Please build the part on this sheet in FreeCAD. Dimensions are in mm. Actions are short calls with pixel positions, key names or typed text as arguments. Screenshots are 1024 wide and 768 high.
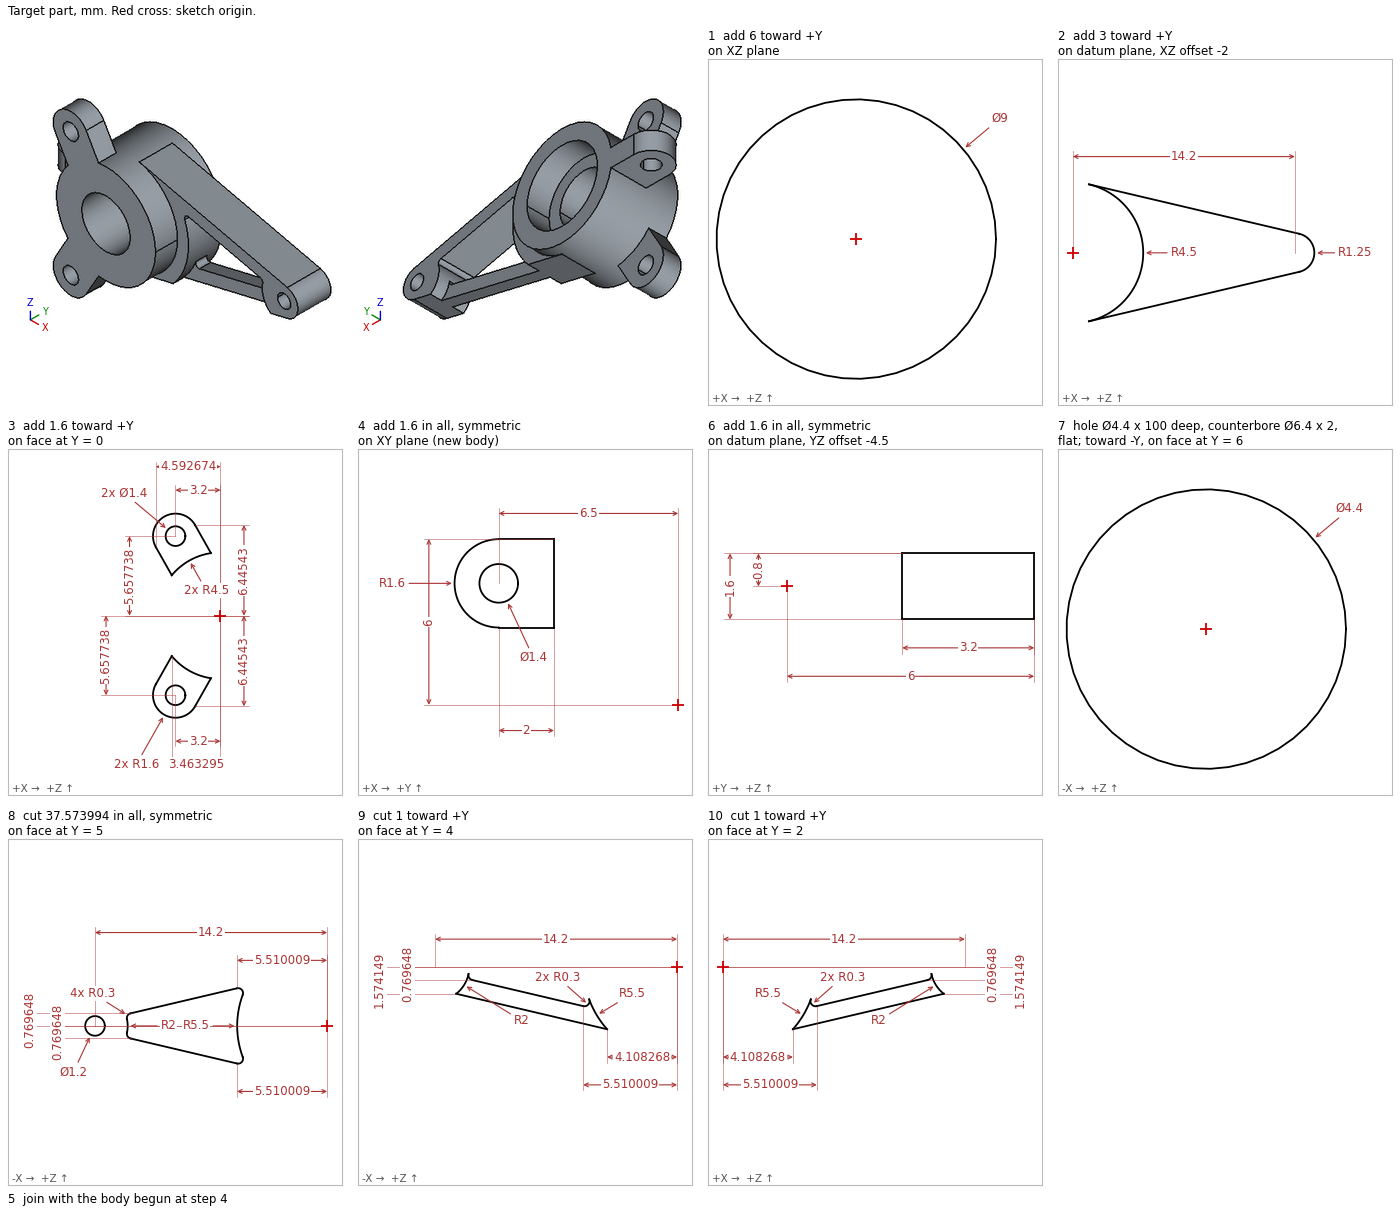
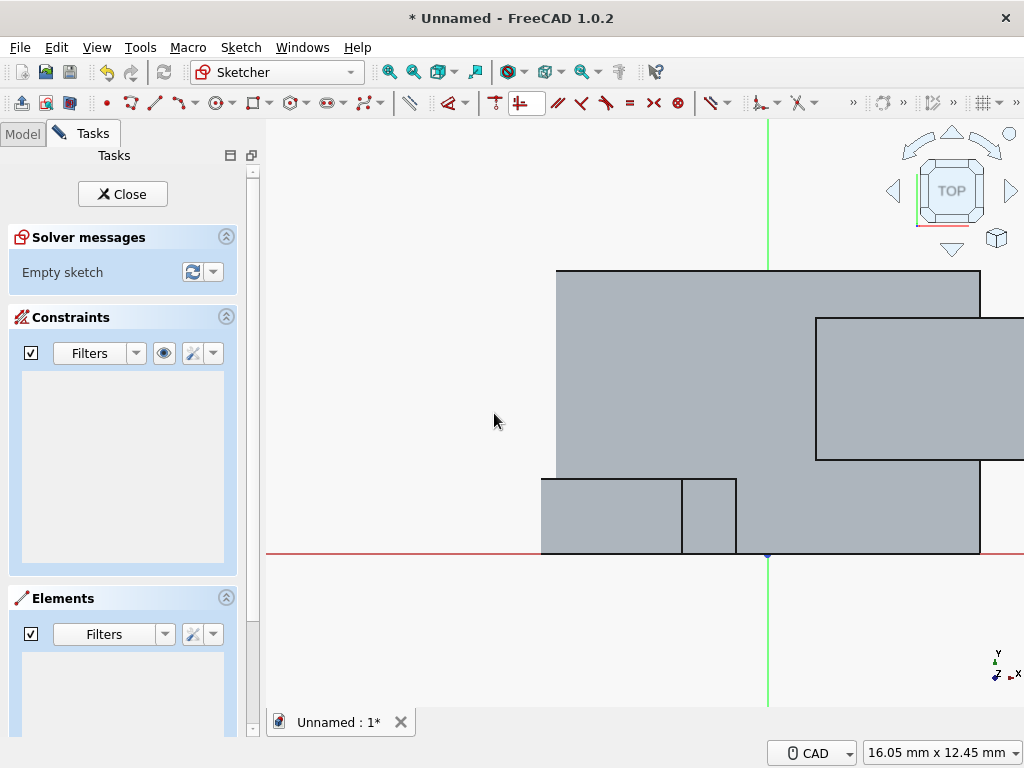
key(g)
key(m)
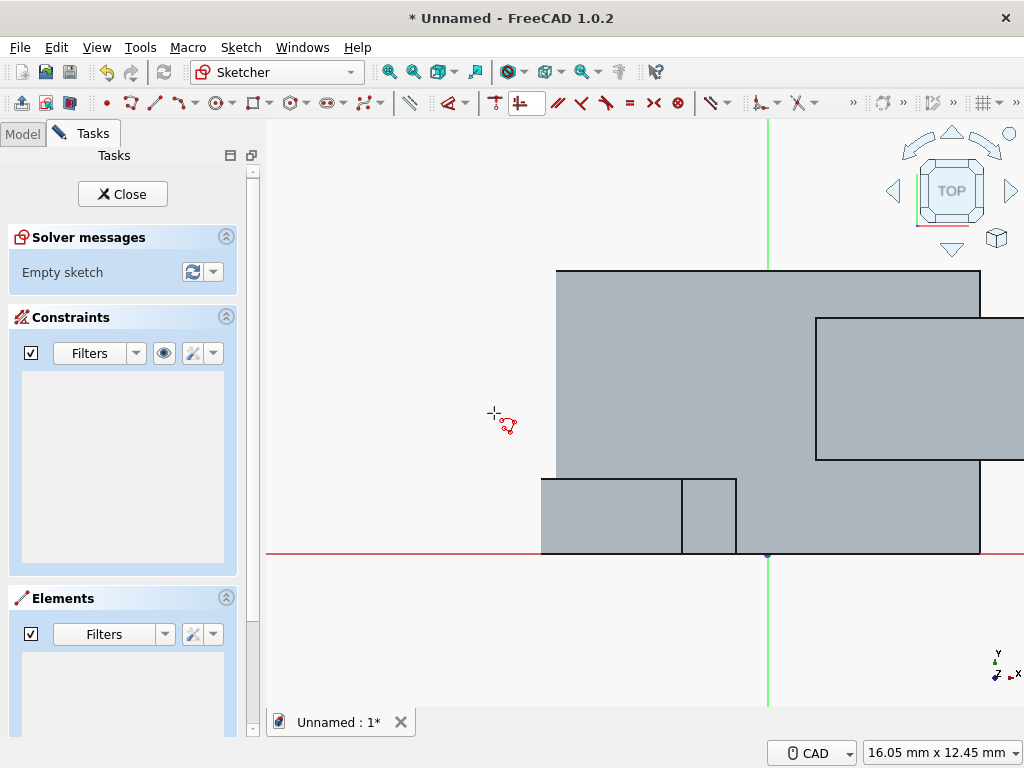
click(461, 422)
click(555, 422)
click(555, 271)
click(461, 271)
right_click(461, 271)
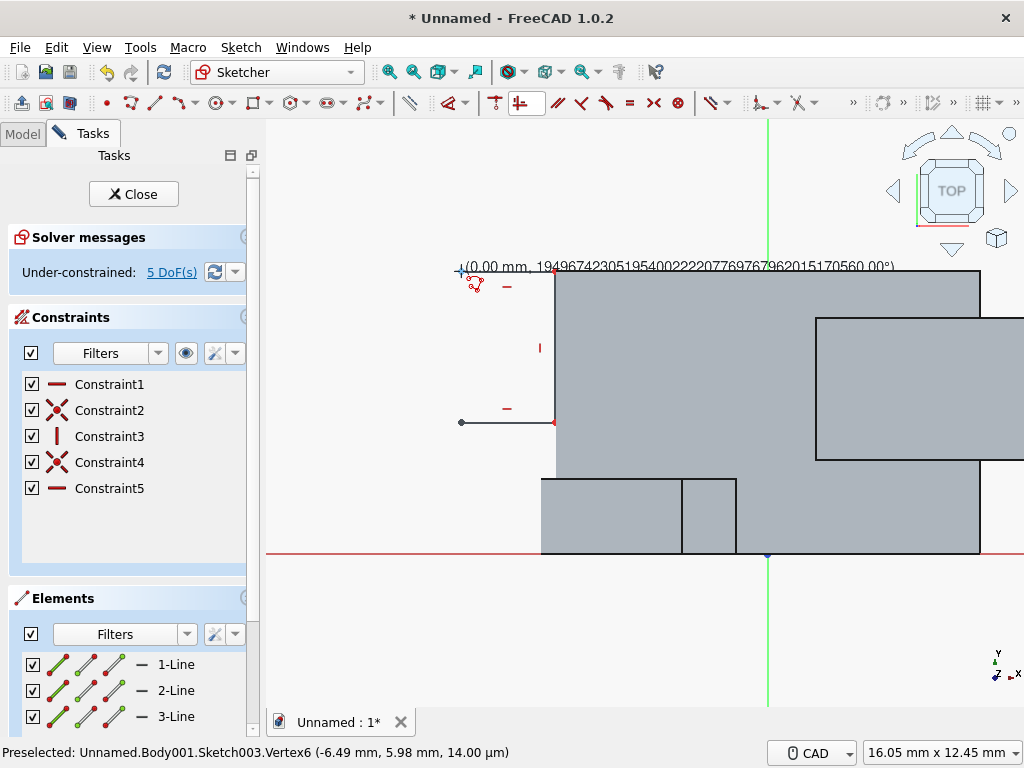
key(g)
key(3)
key(a)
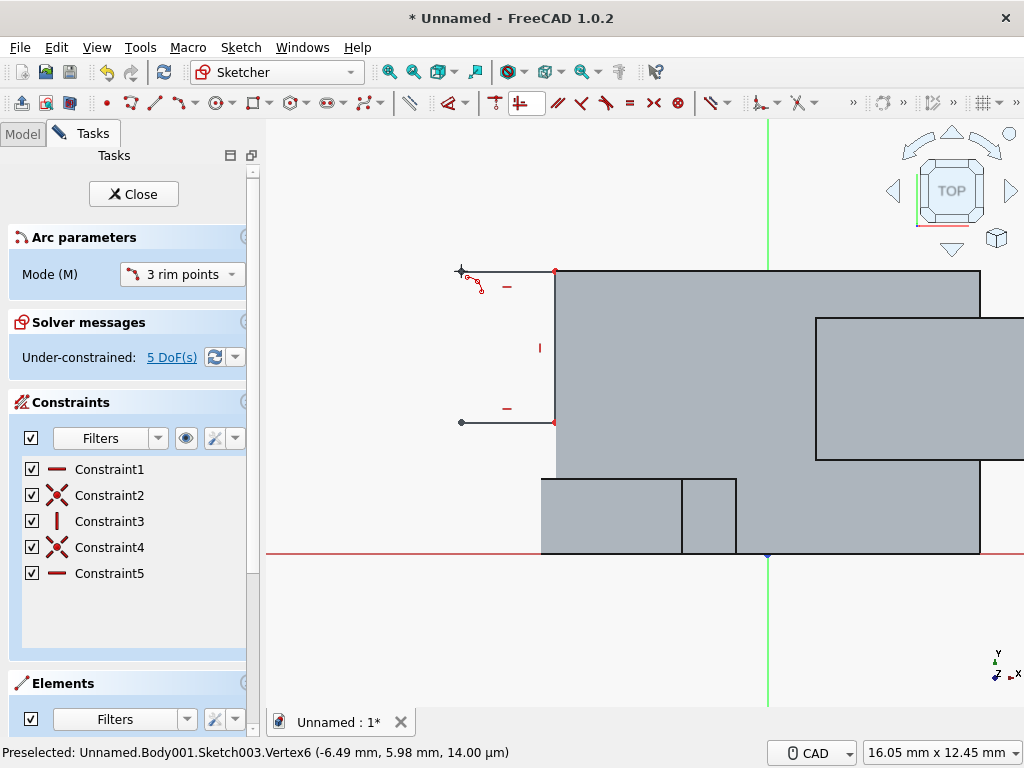
click(461, 272)
click(461, 423)
click(385, 346)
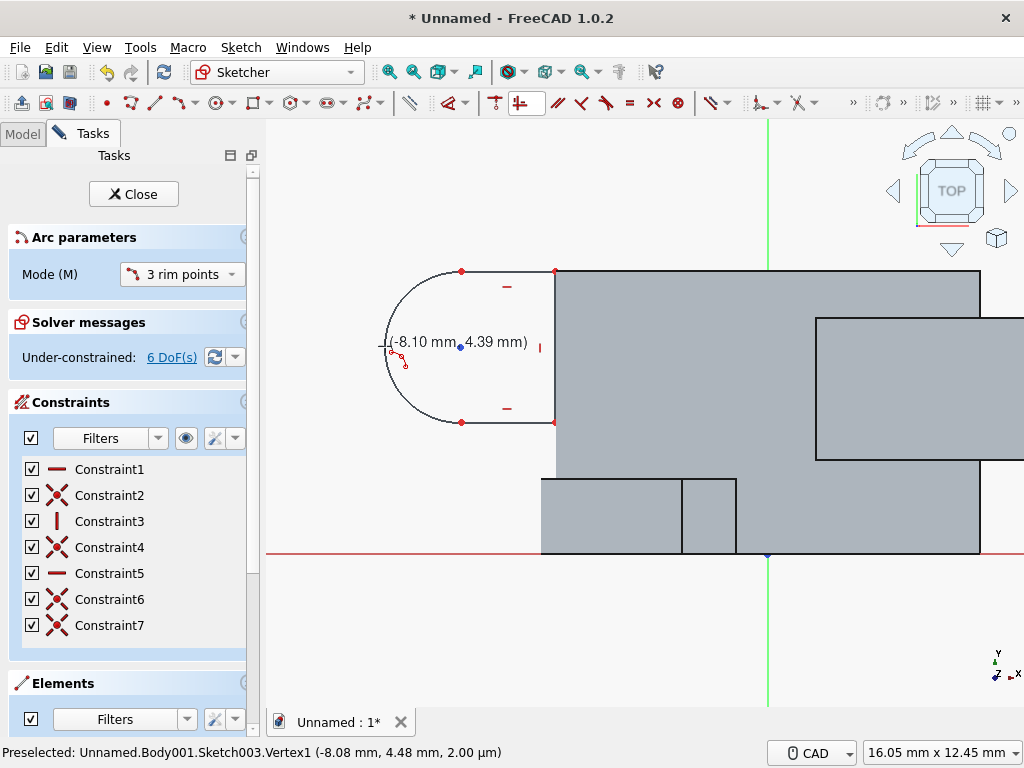
key(g)
key(c)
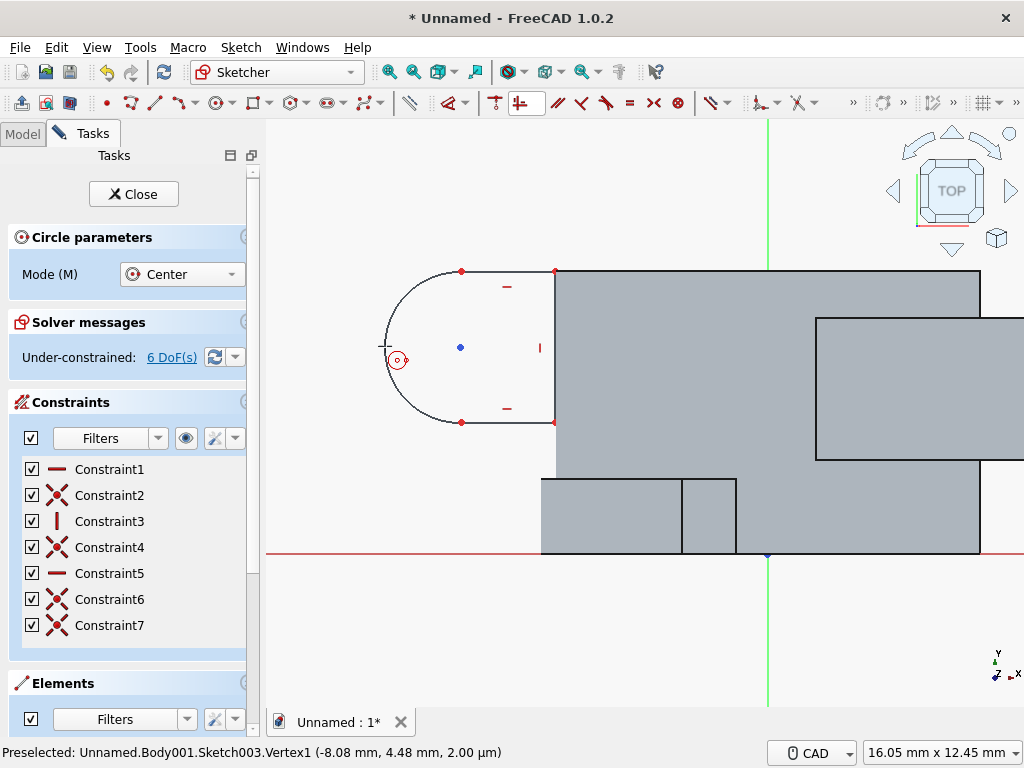
click(461, 346)
click(484, 323)
key(Escape)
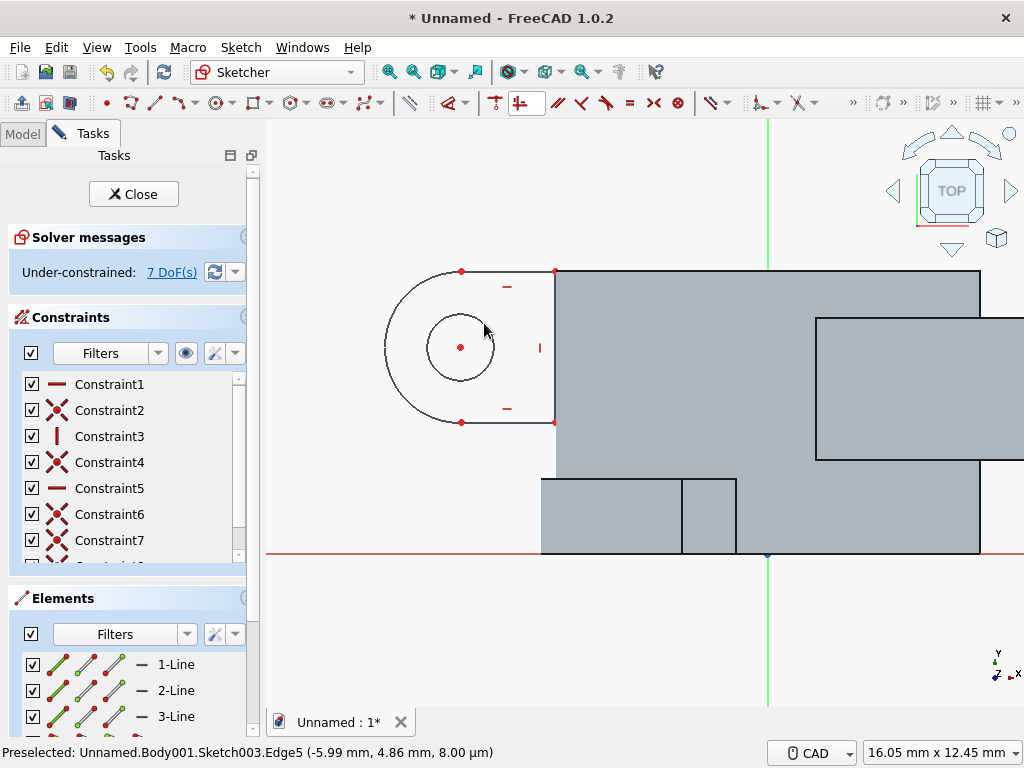
click(489, 423)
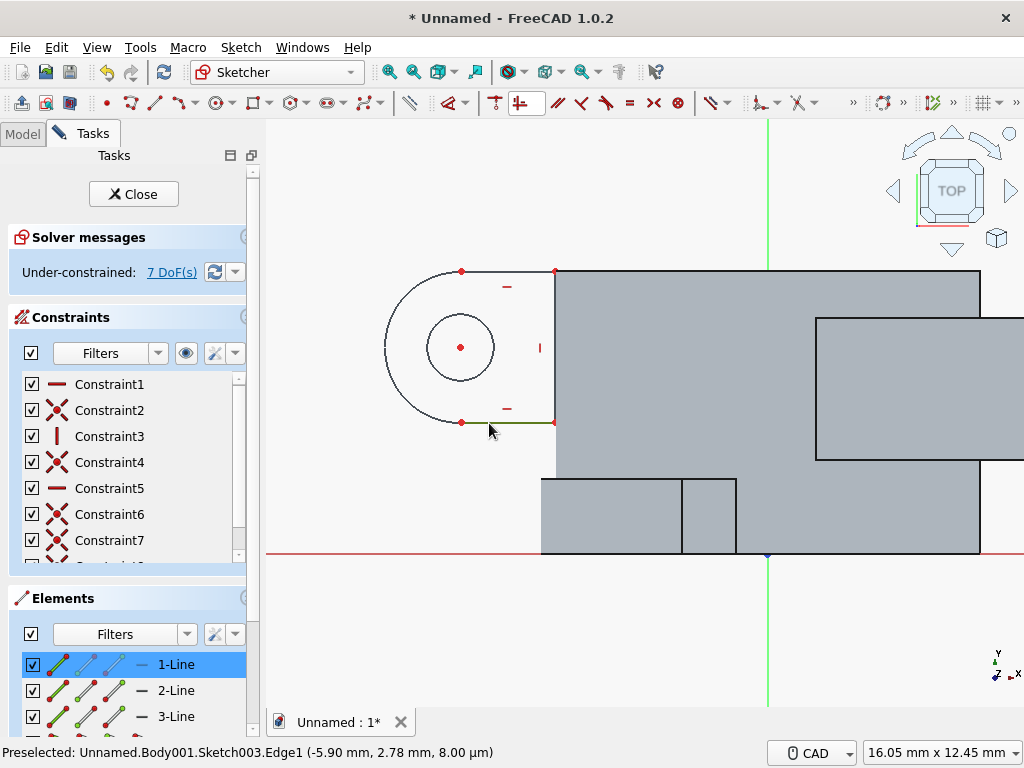
click(400, 303)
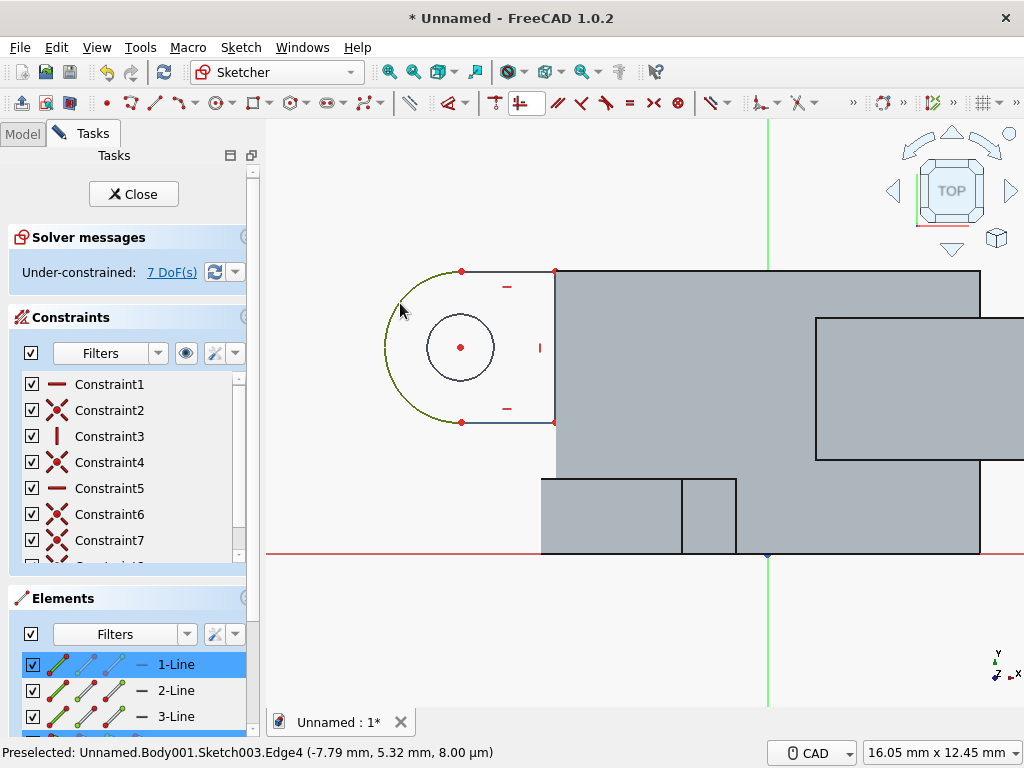
click(606, 104)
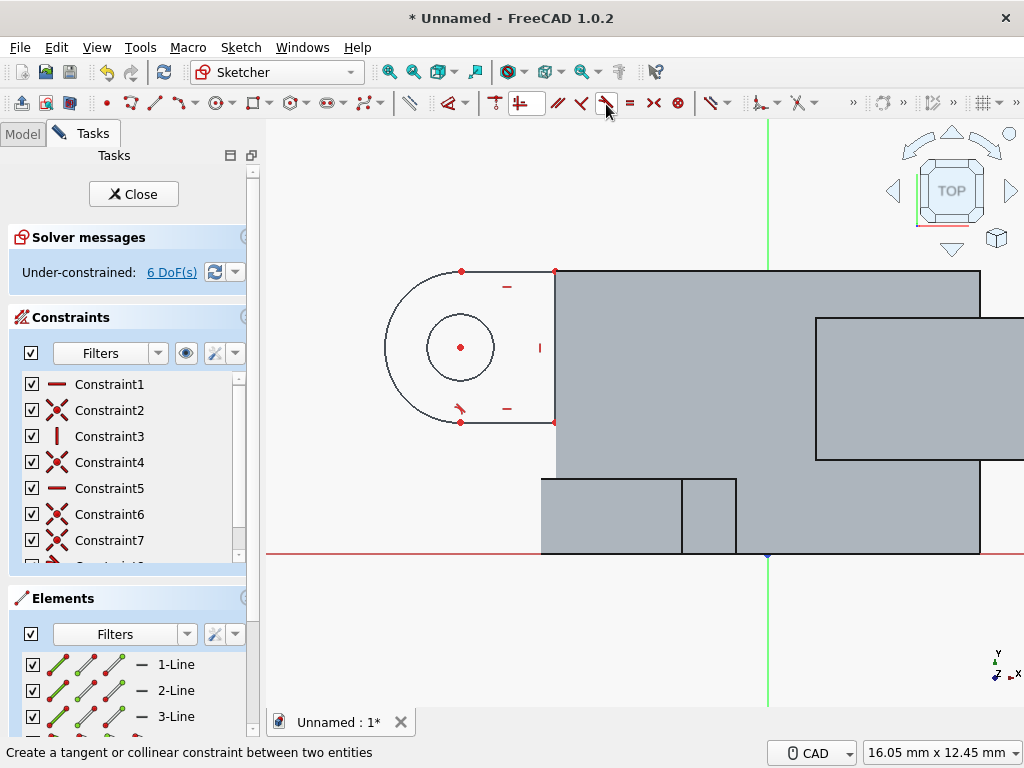
click(527, 272)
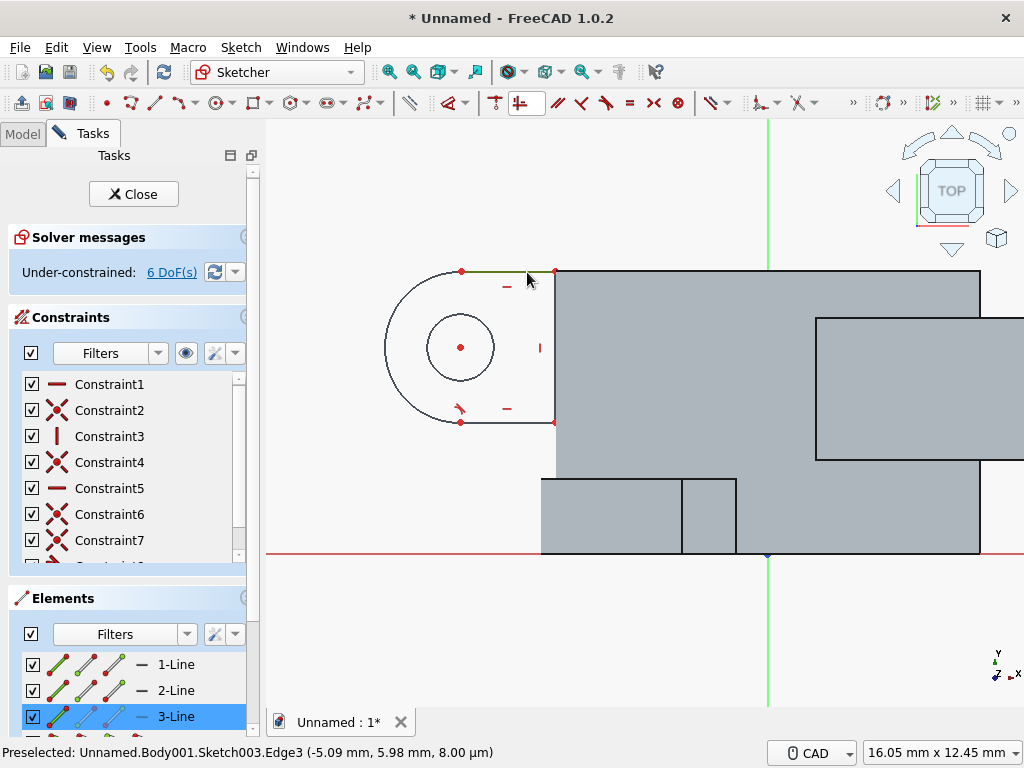
click(400, 303)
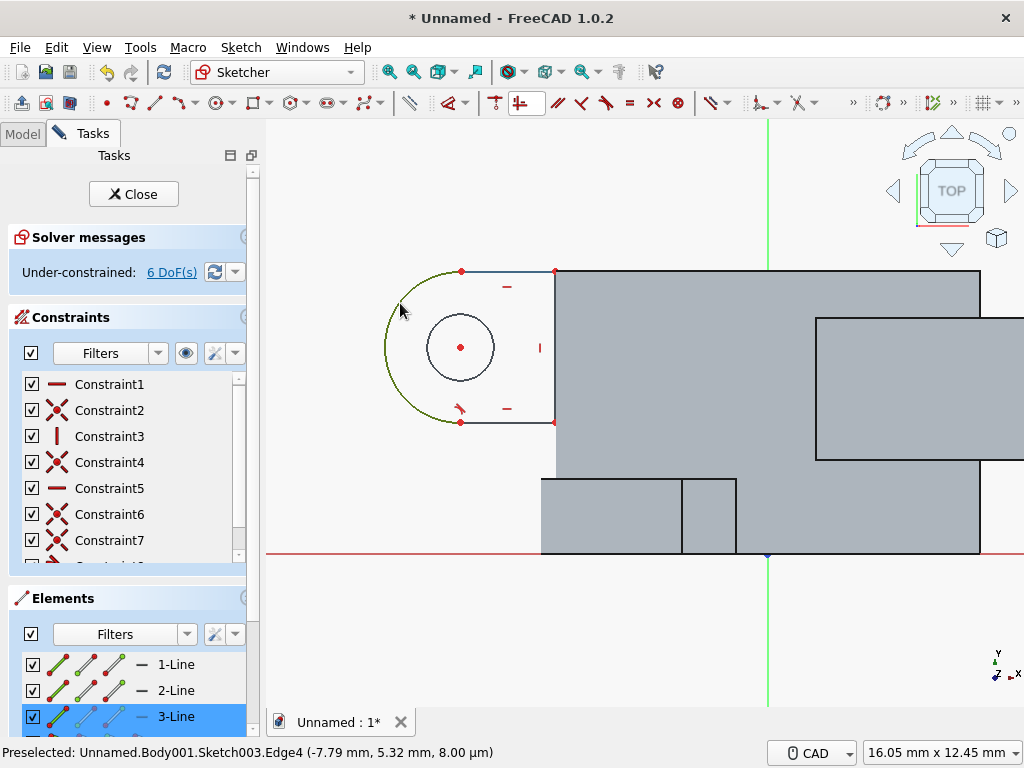
key(t)